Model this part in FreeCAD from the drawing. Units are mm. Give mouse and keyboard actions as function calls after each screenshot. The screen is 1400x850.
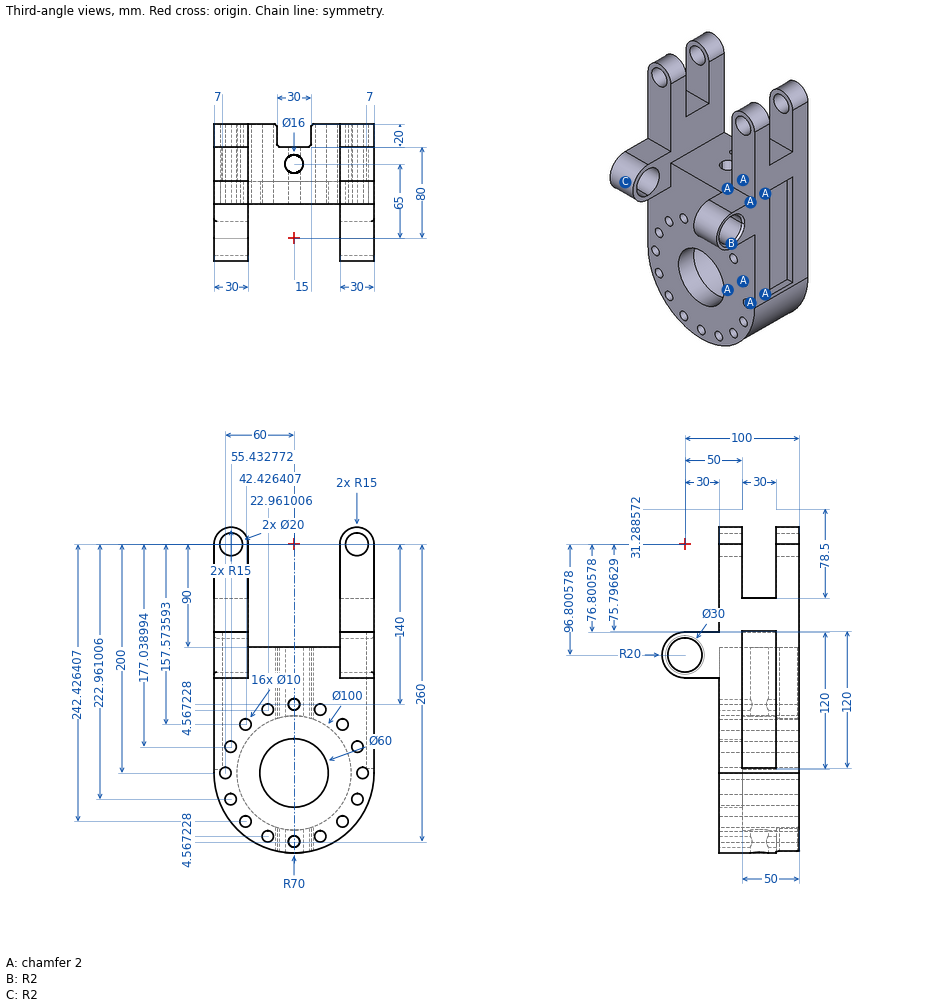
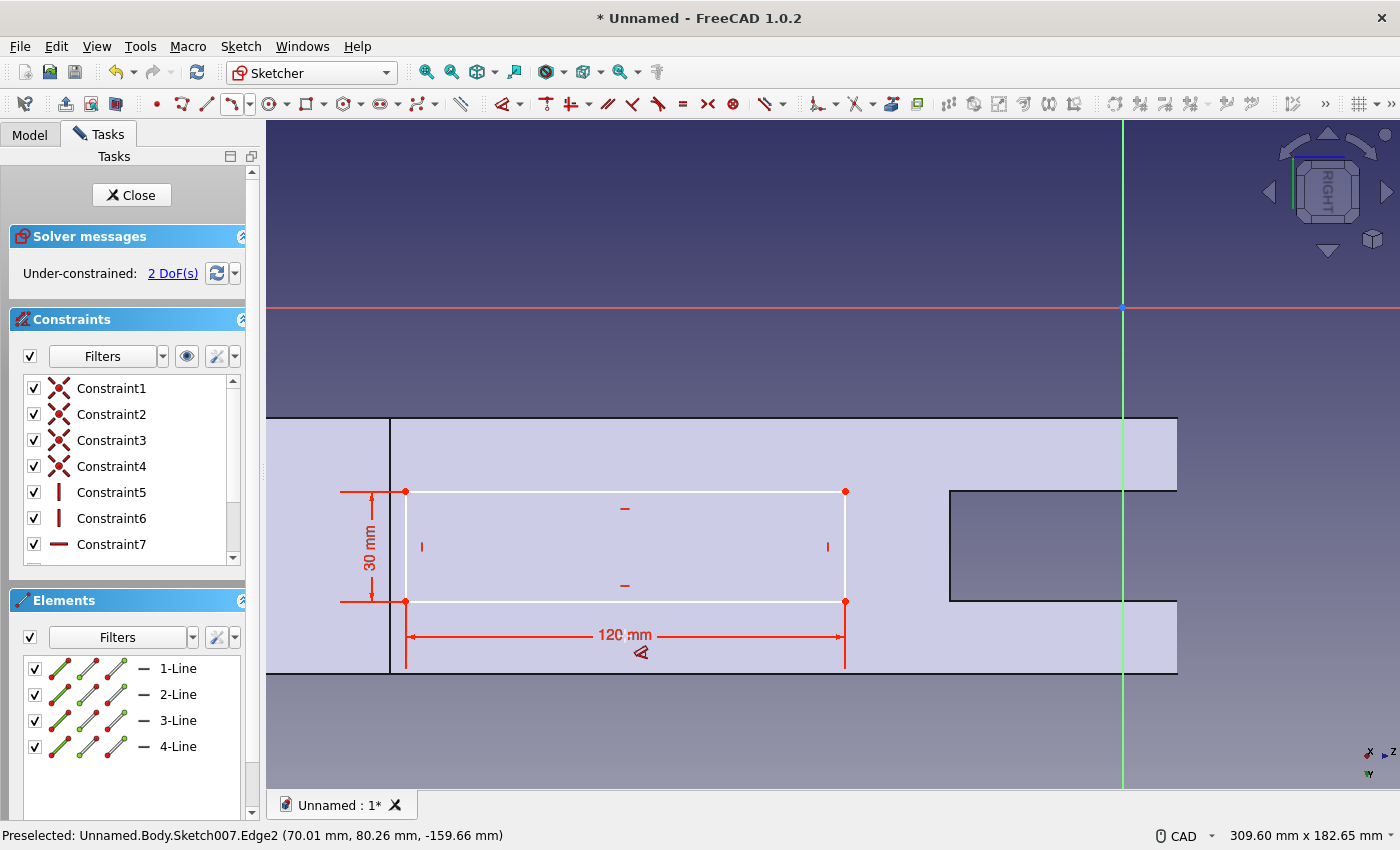
click(406, 492)
click(1157, 400)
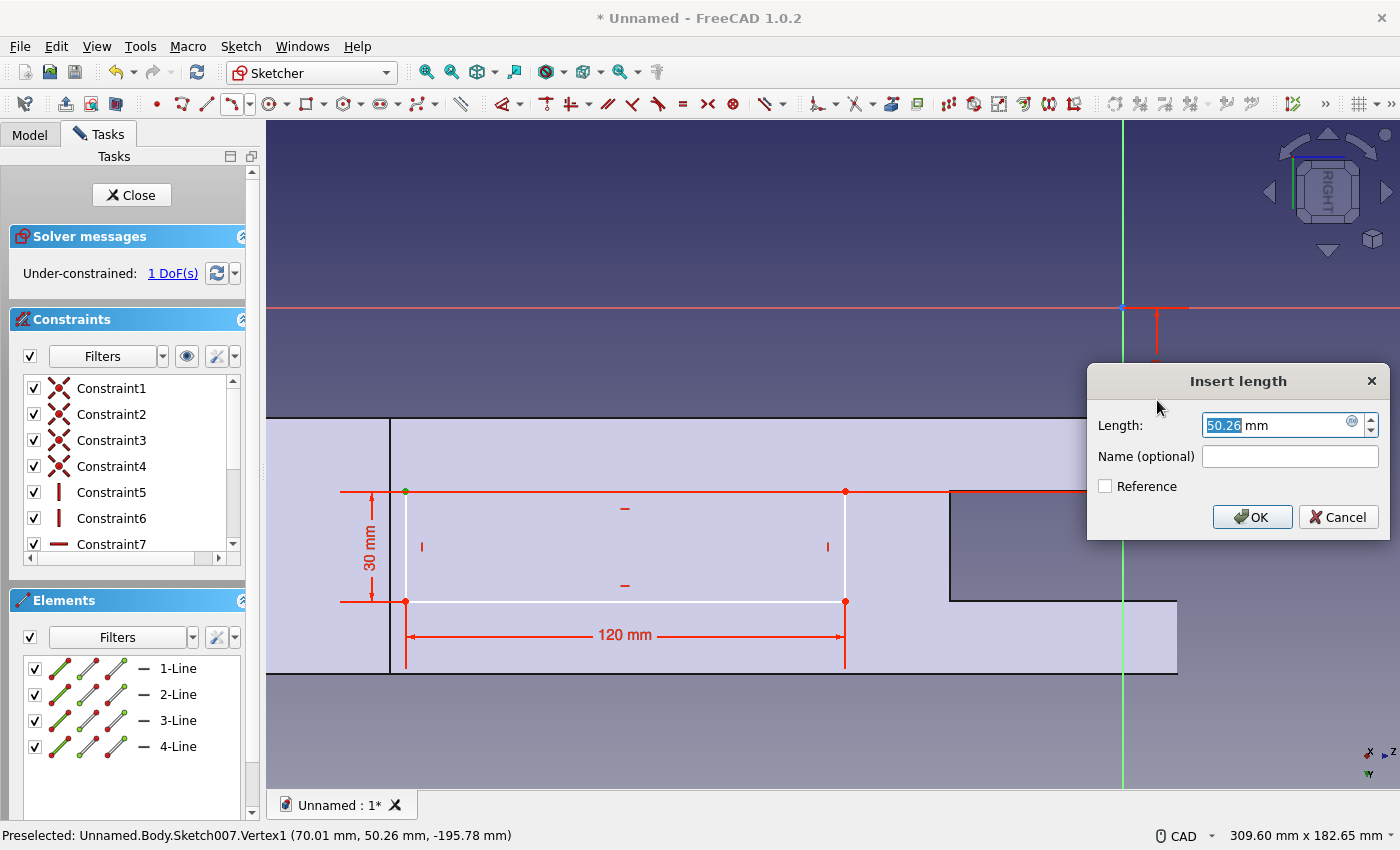
text(50)
key(Return)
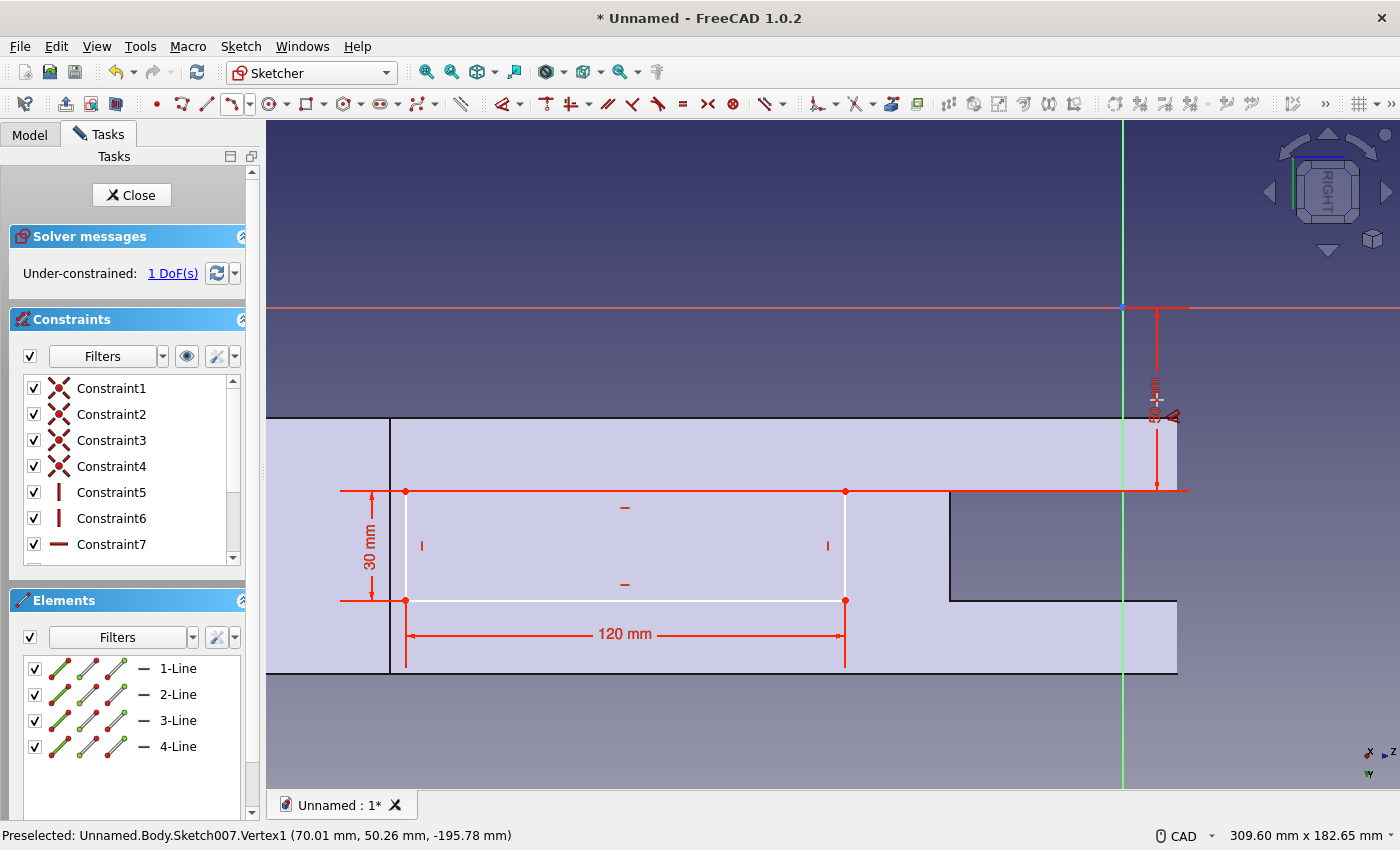
click(845, 601)
click(984, 635)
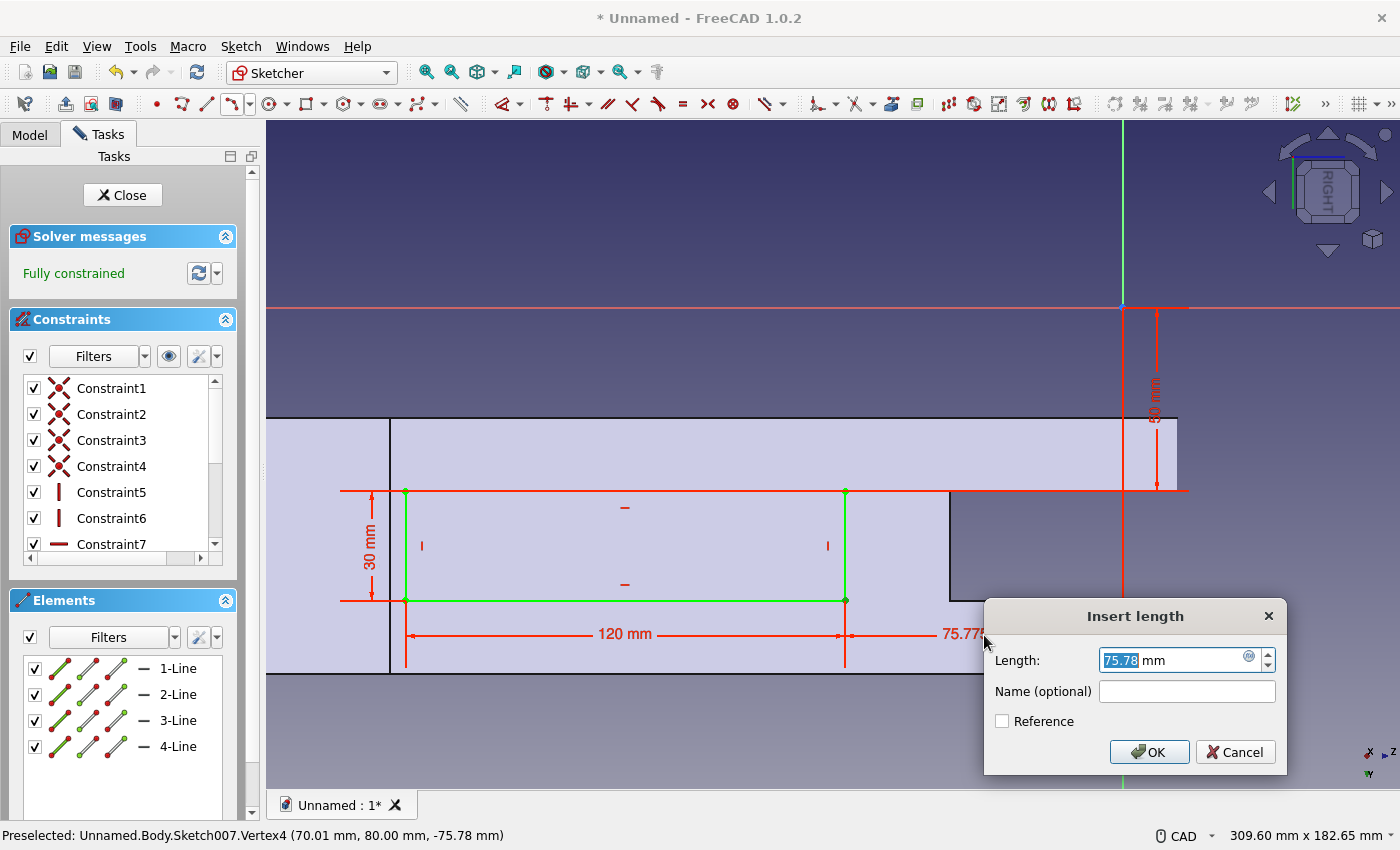
text(75.796629)
key(Return)
key(Escape)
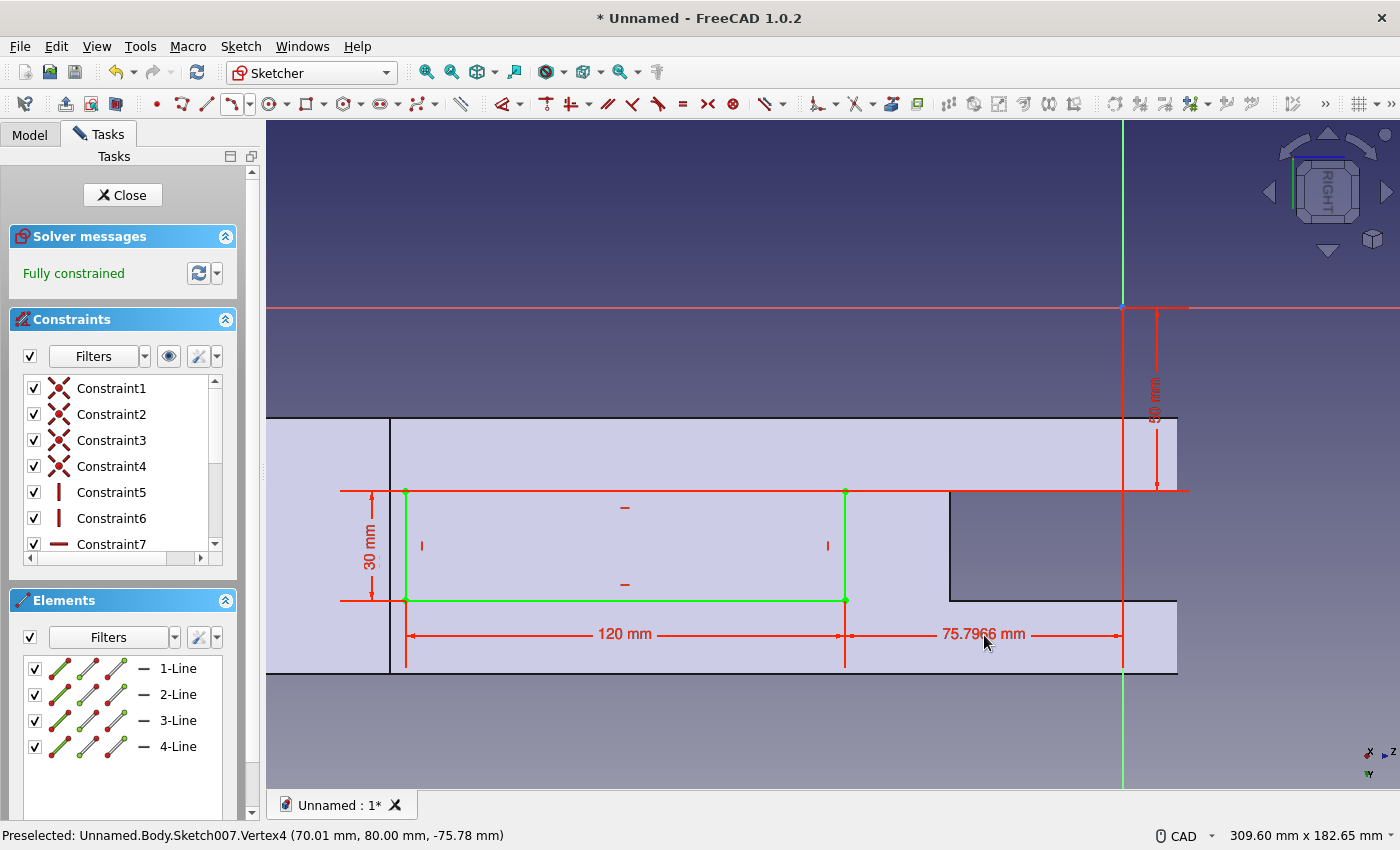
click(123, 195)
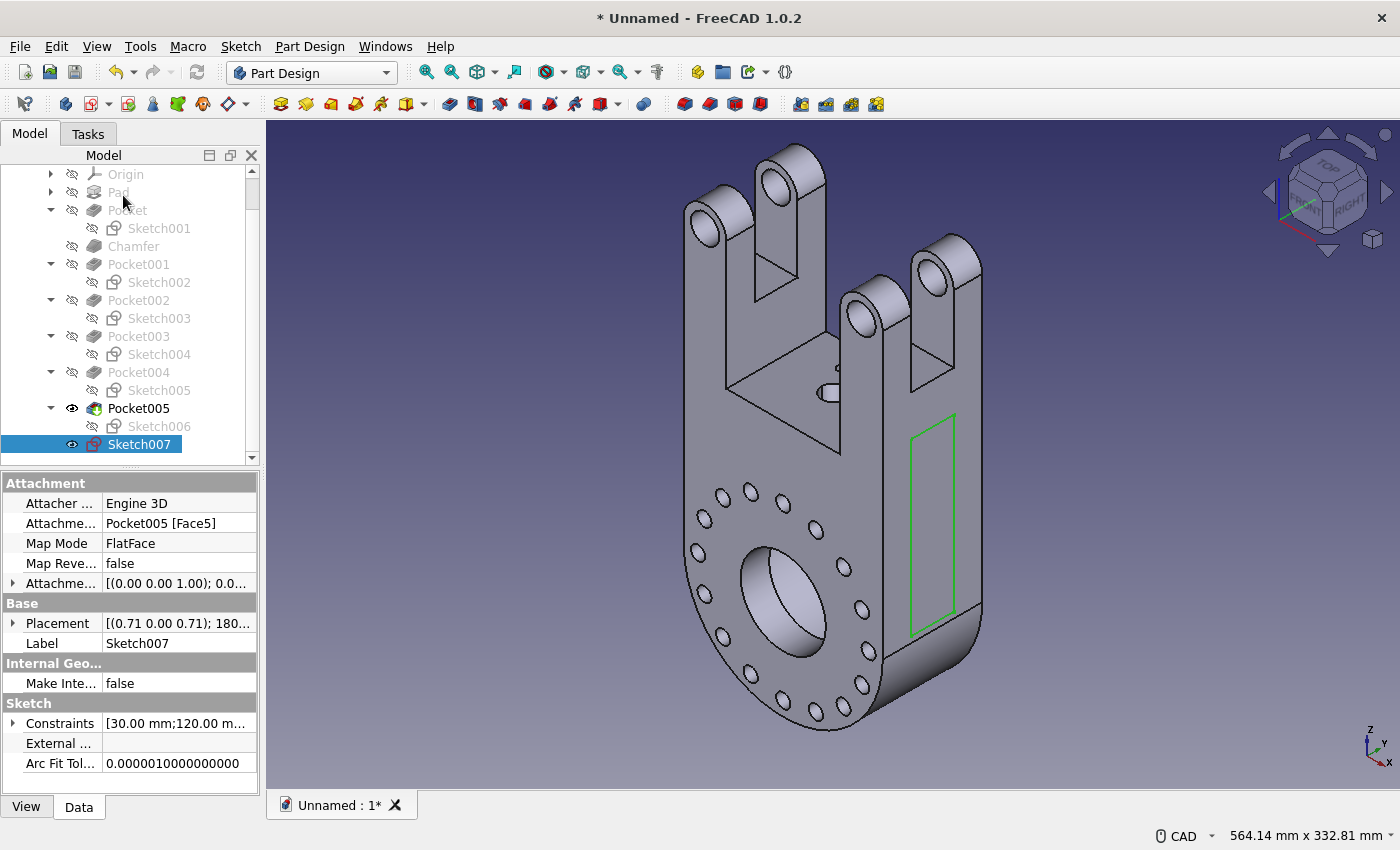
click(450, 104)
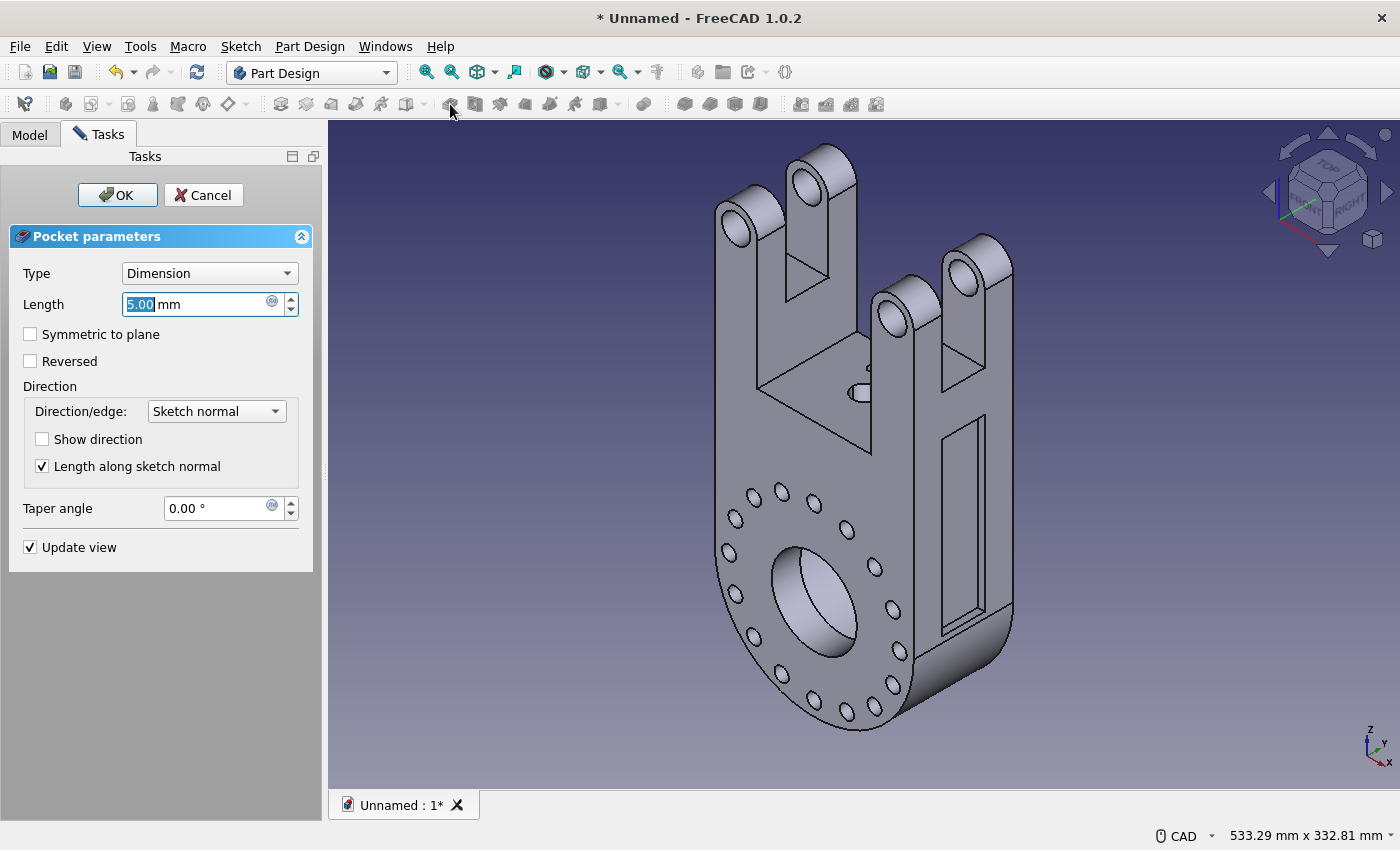
text(7)
key(Tab)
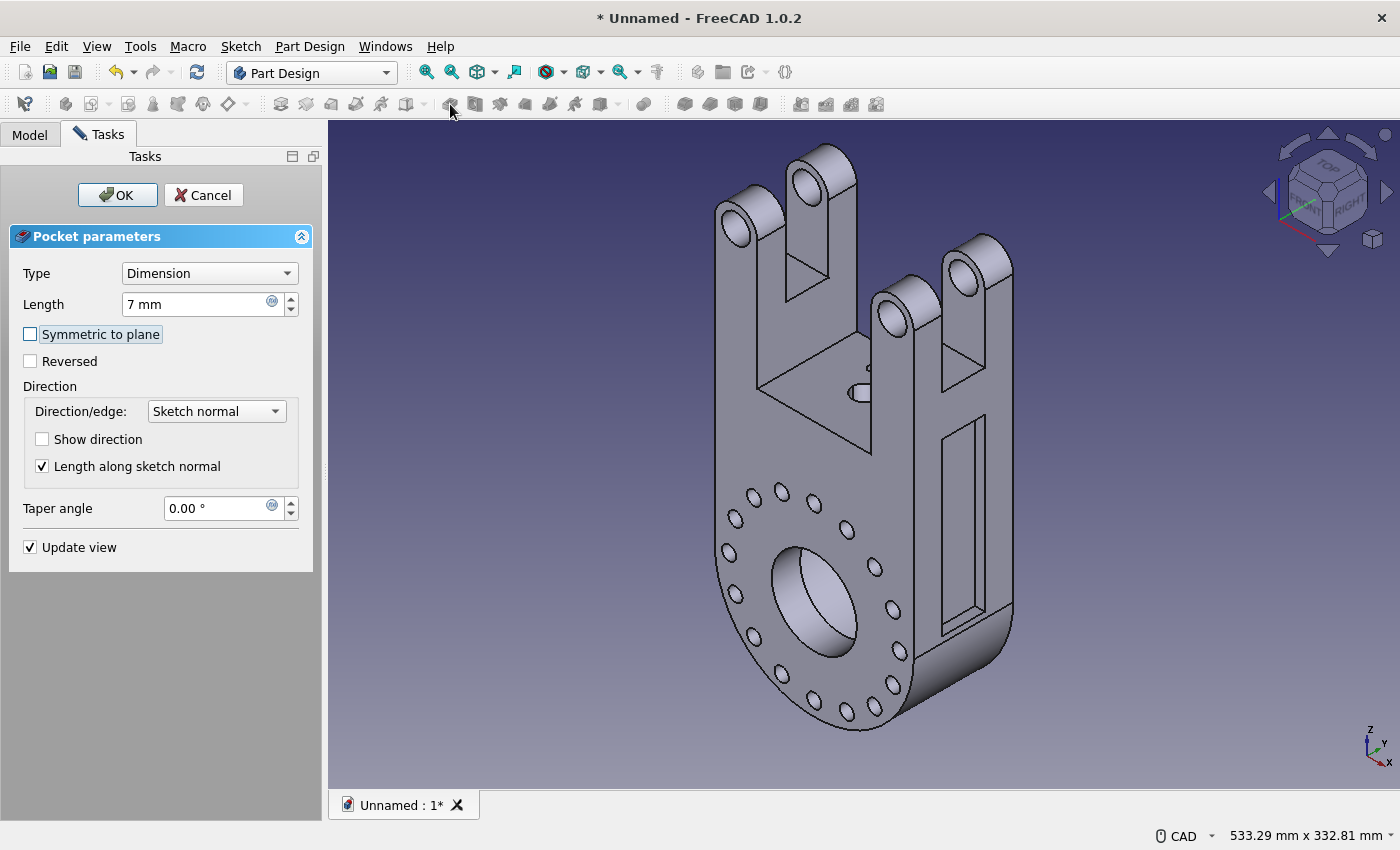
click(118, 195)